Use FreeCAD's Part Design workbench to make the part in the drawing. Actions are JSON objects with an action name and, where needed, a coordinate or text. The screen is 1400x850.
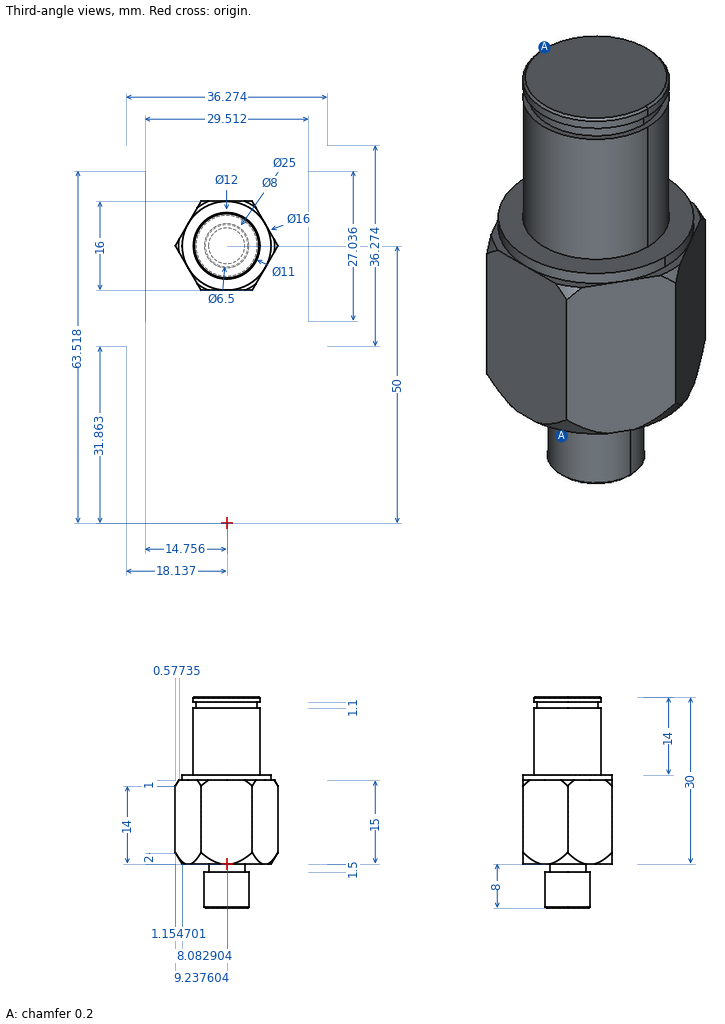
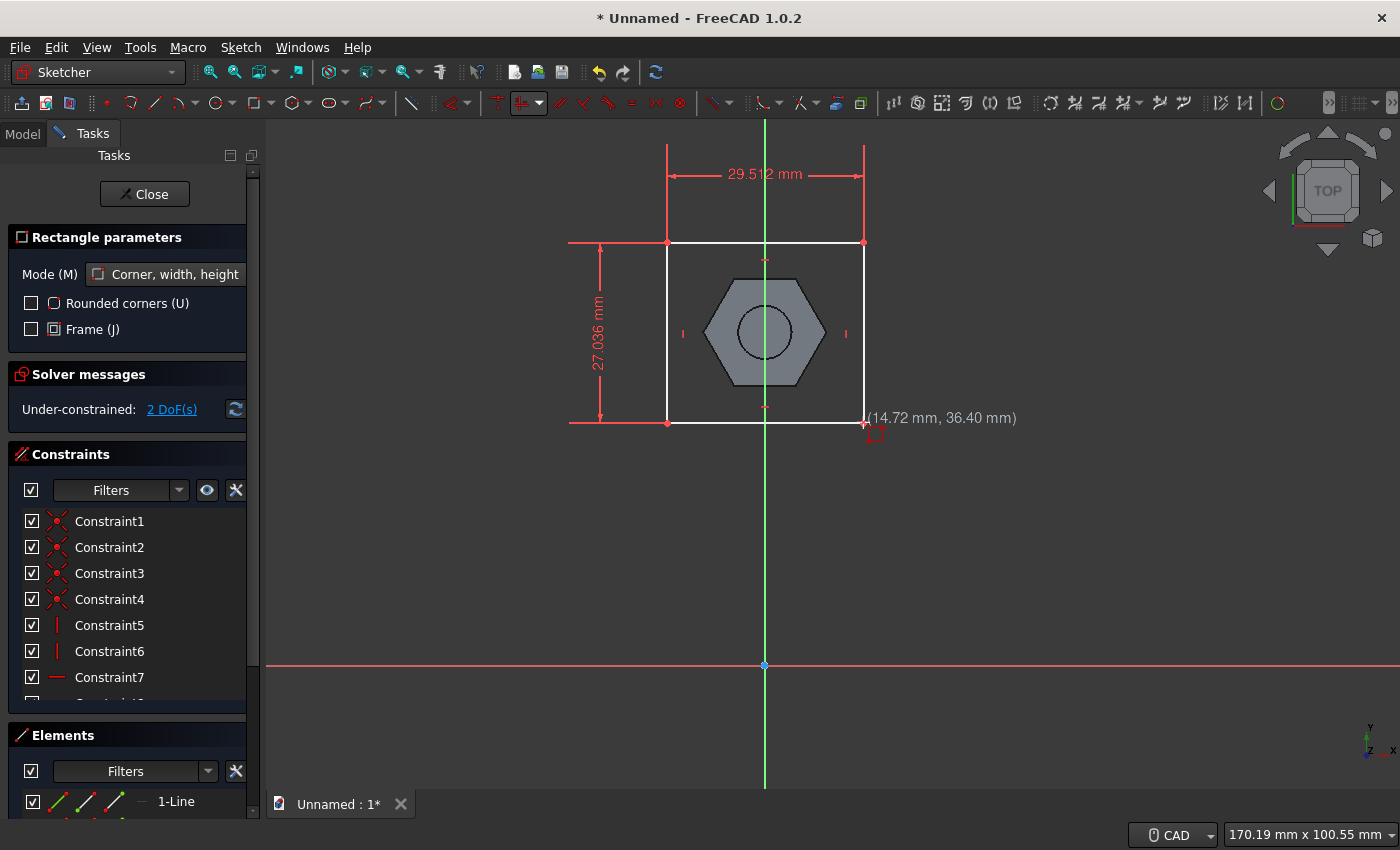
{"action": "left_click", "coordinate": [216, 104]}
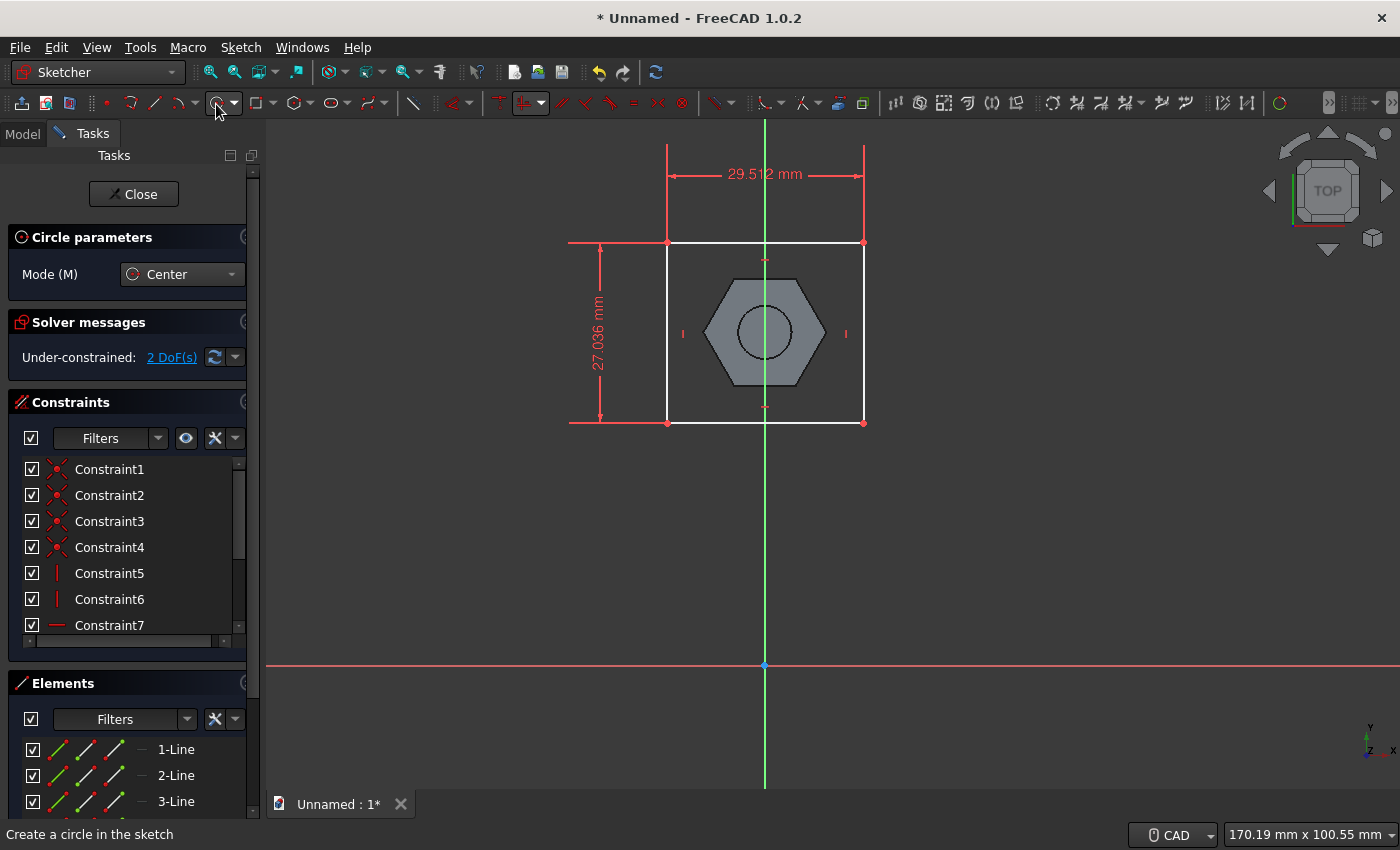
{"action": "left_click", "coordinate": [765, 332]}
{"action": "mouse_move", "coordinate": [780, 317]}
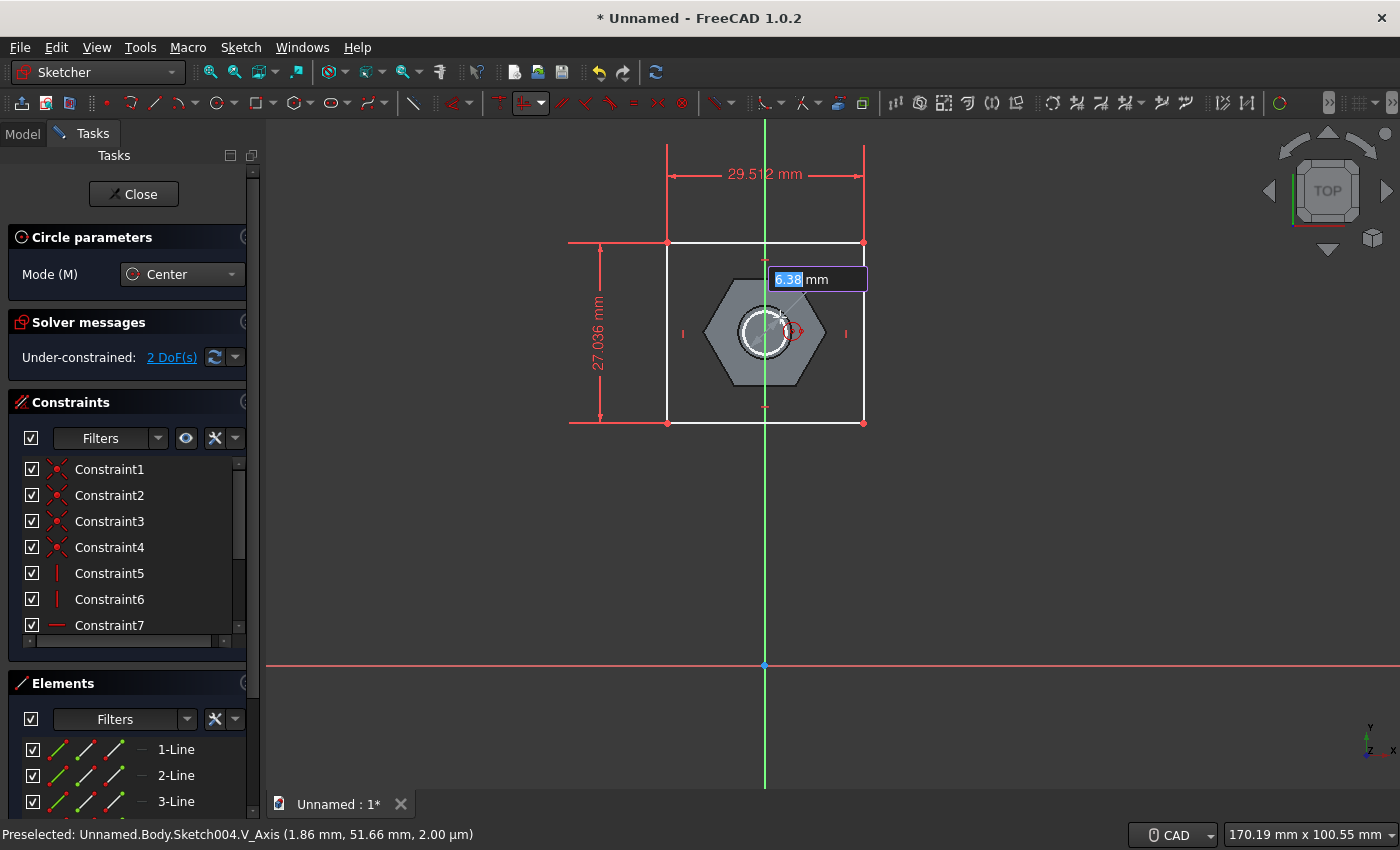
{"action": "type", "text": "6.5"}
{"action": "key", "text": "Return"}
{"action": "key", "text": "Escape"}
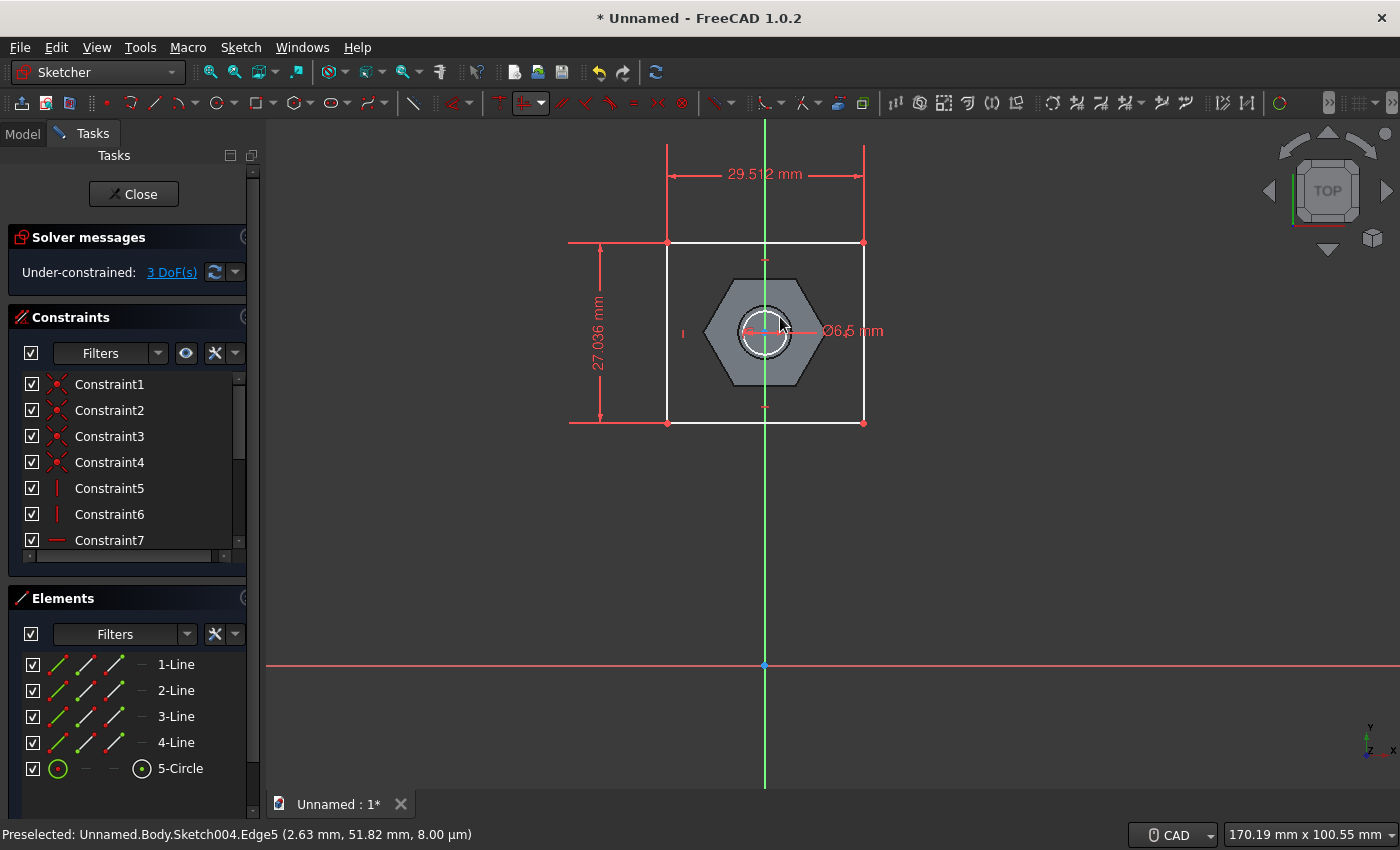
{"action": "left_click", "coordinate": [452, 104]}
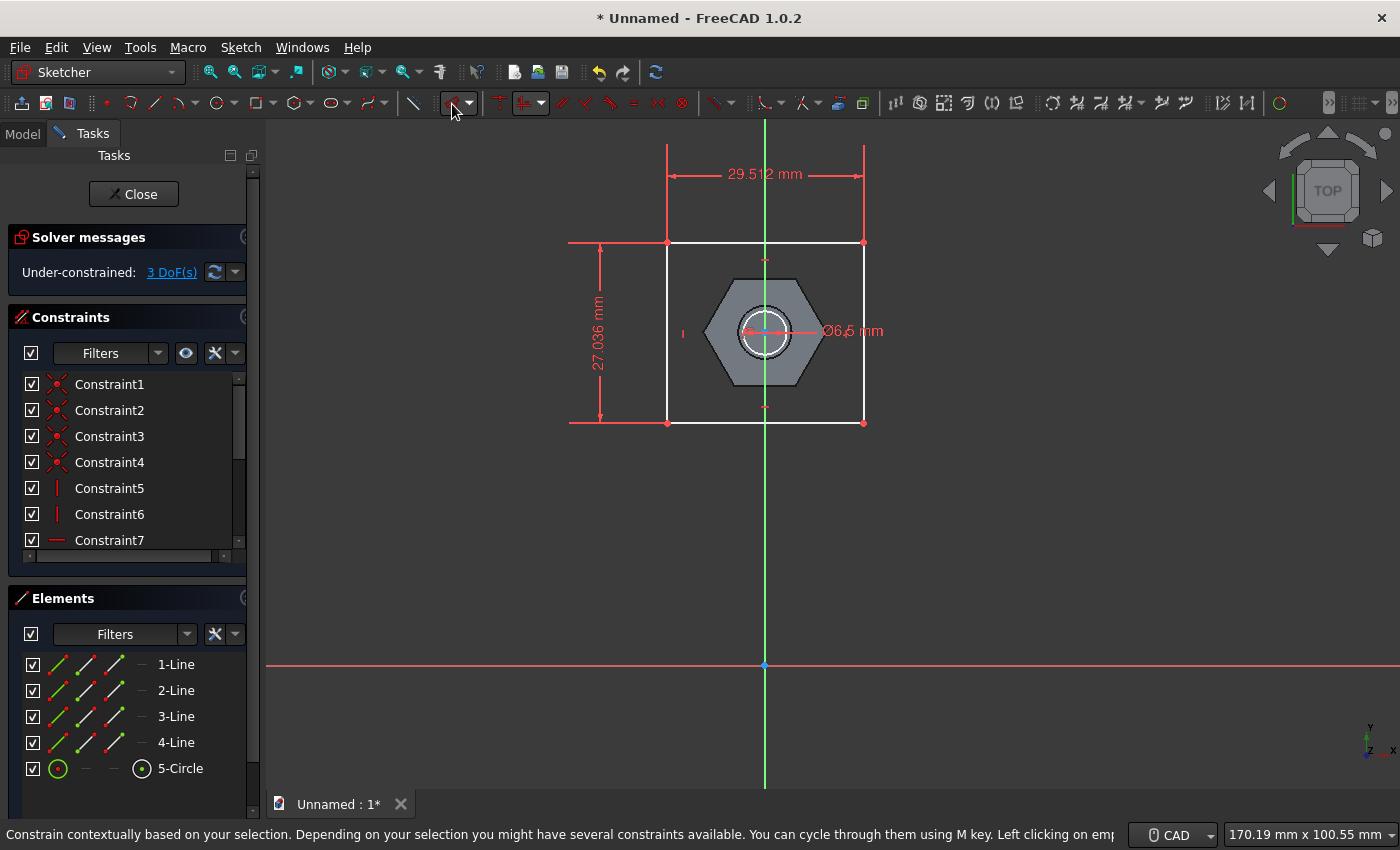
{"action": "left_click", "coordinate": [765, 333]}
{"action": "left_click", "coordinate": [799, 499]}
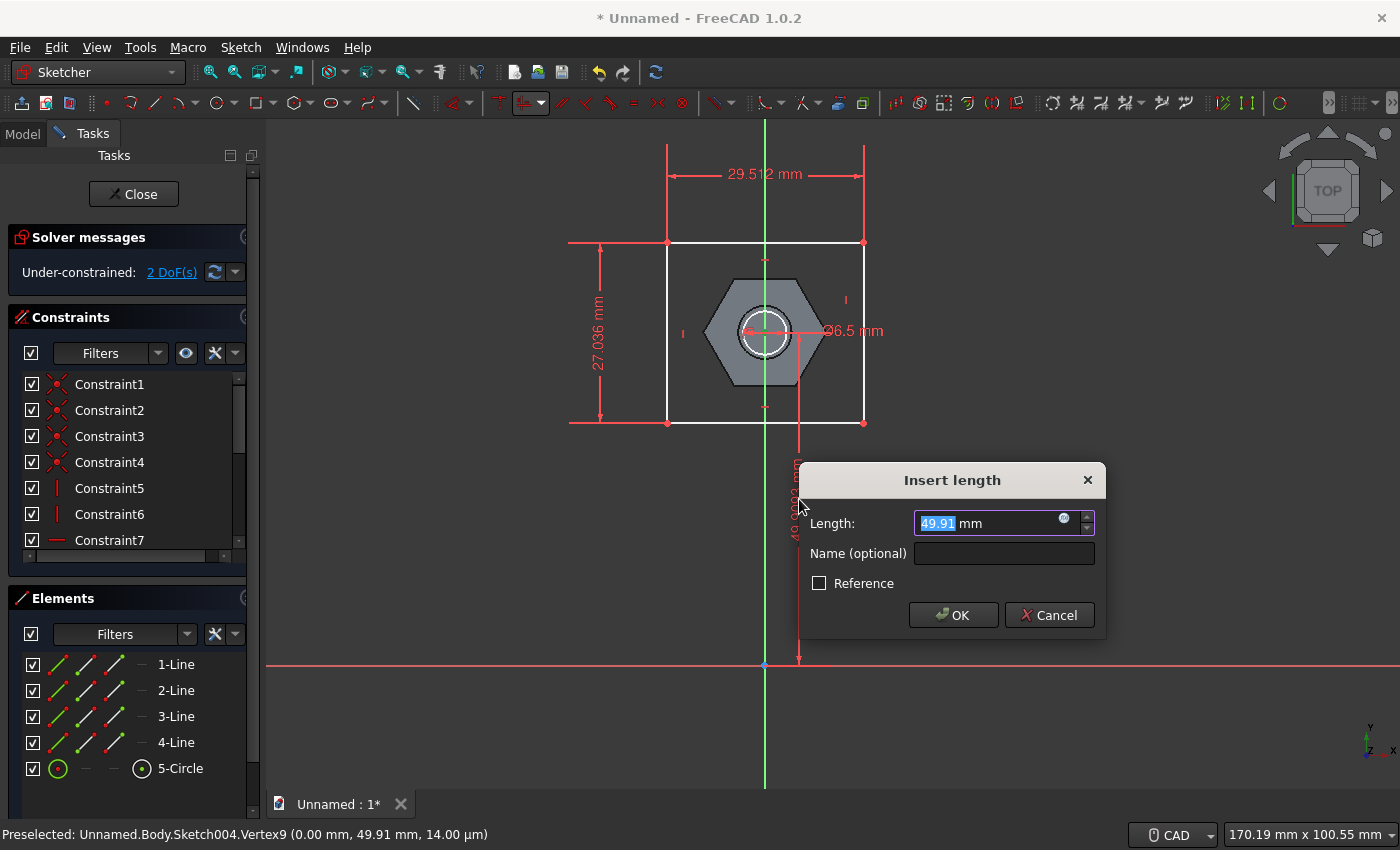
{"action": "type", "text": "50"}
{"action": "key", "text": "Return"}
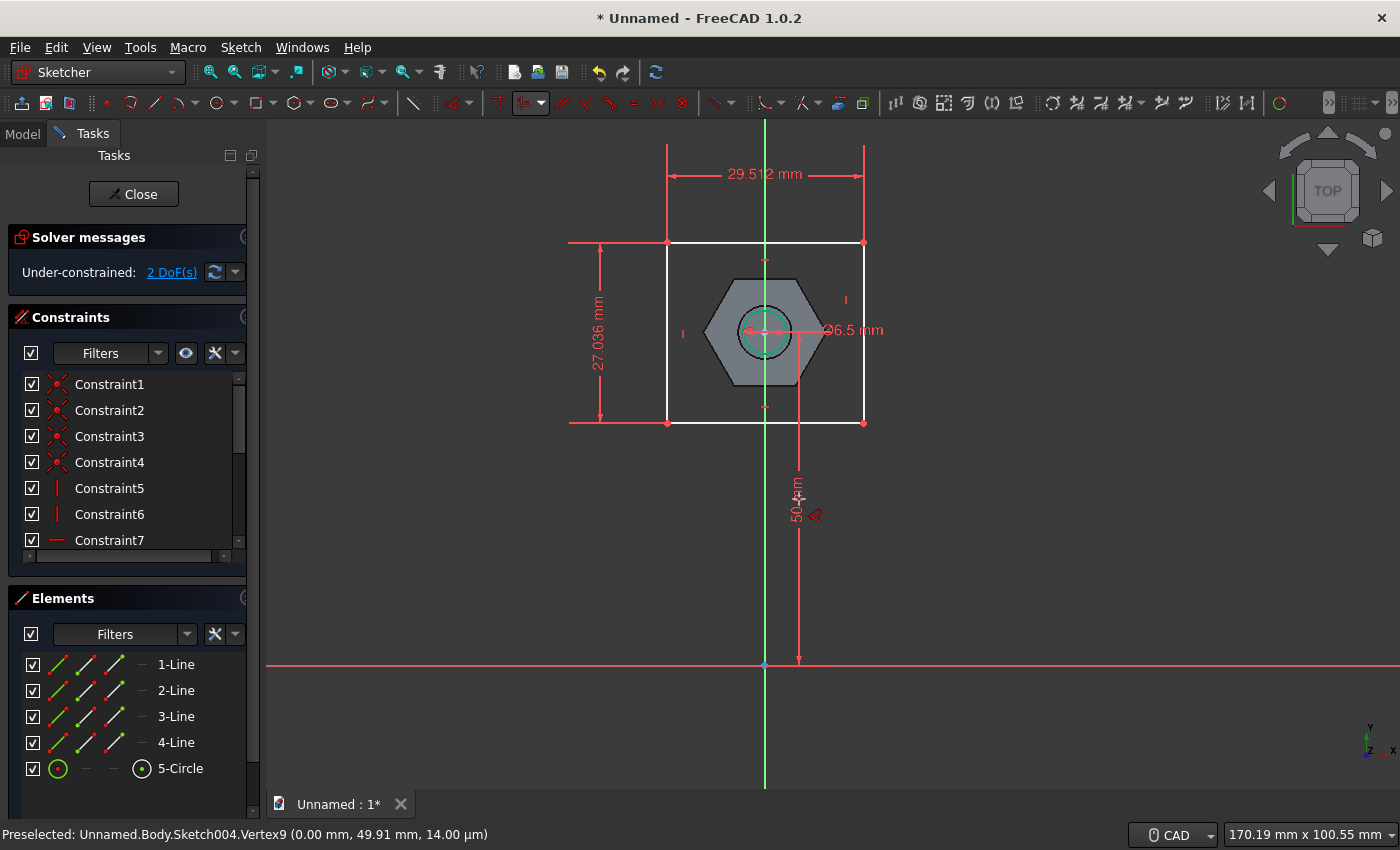
{"action": "left_click", "coordinate": [667, 243]}
{"action": "left_click", "coordinate": [716, 700]}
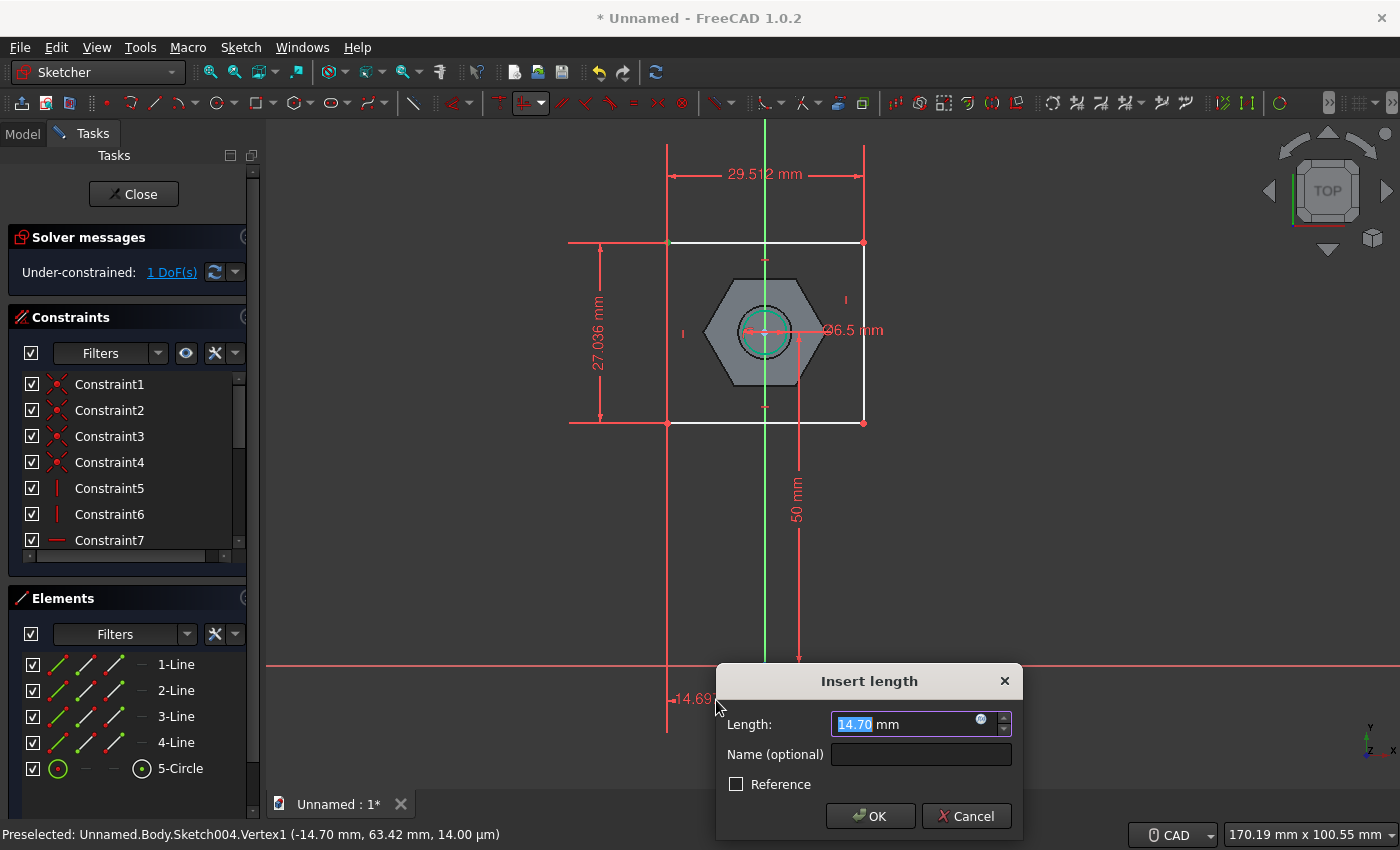
{"action": "type", "text": "14.756"}
{"action": "key", "text": "Return"}